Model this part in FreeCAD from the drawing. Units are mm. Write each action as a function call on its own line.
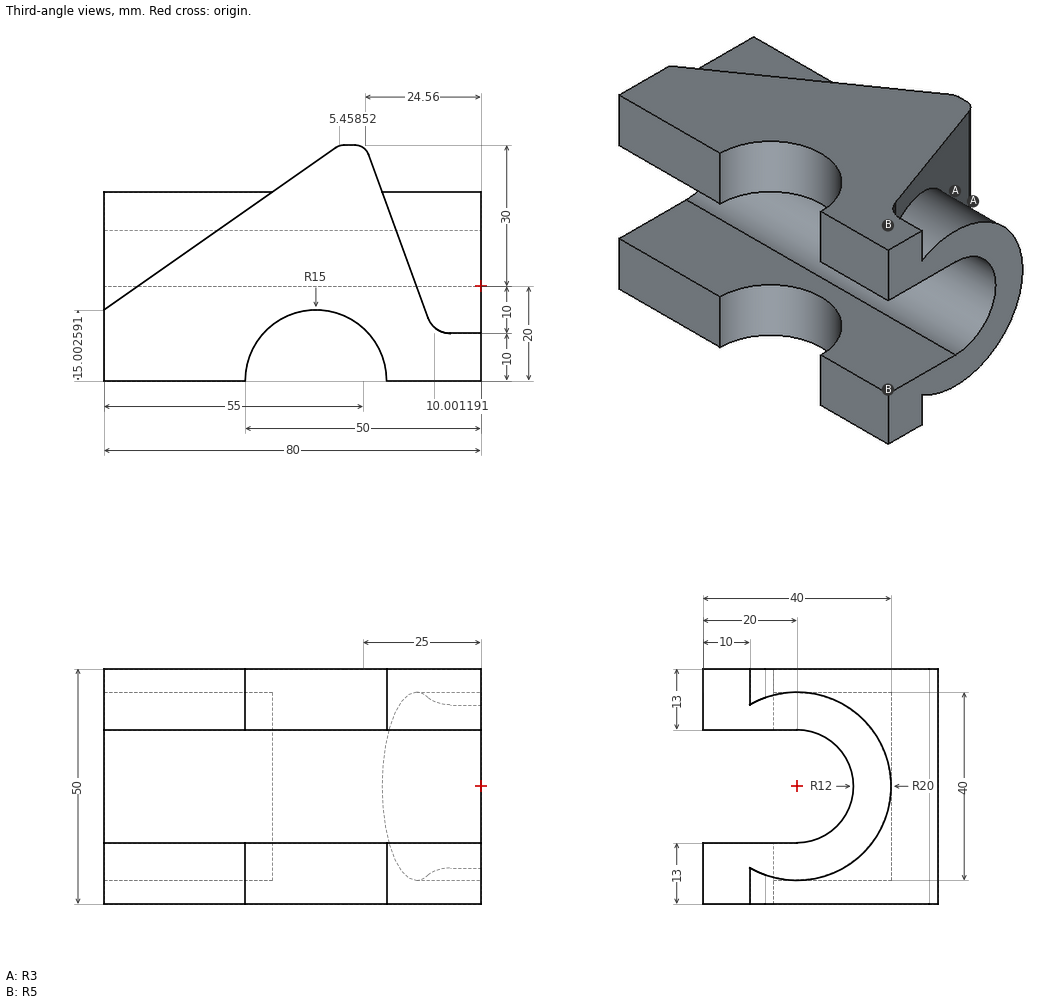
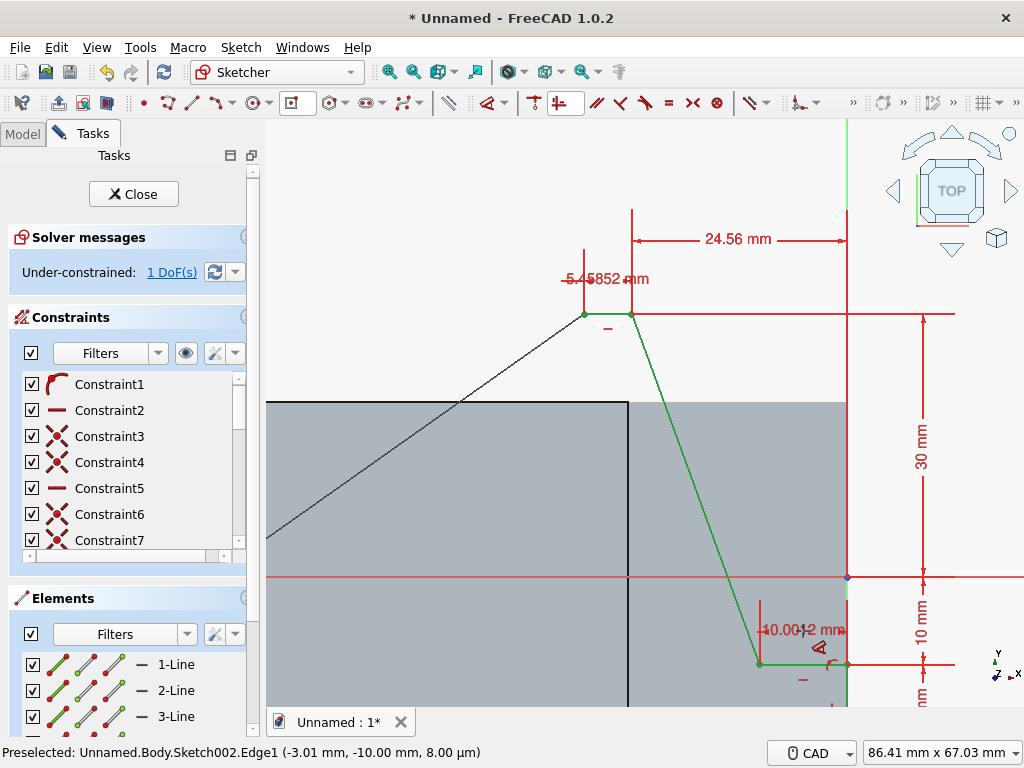
scroll(674, 267, down, 3)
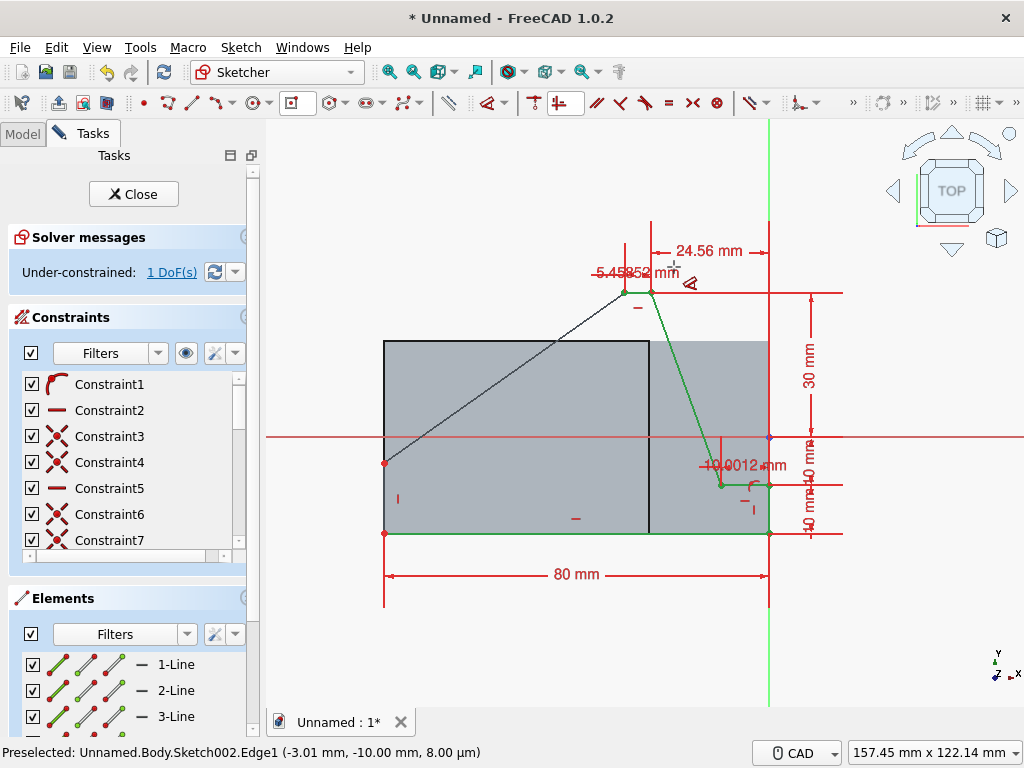
click(384, 484)
click(350, 498)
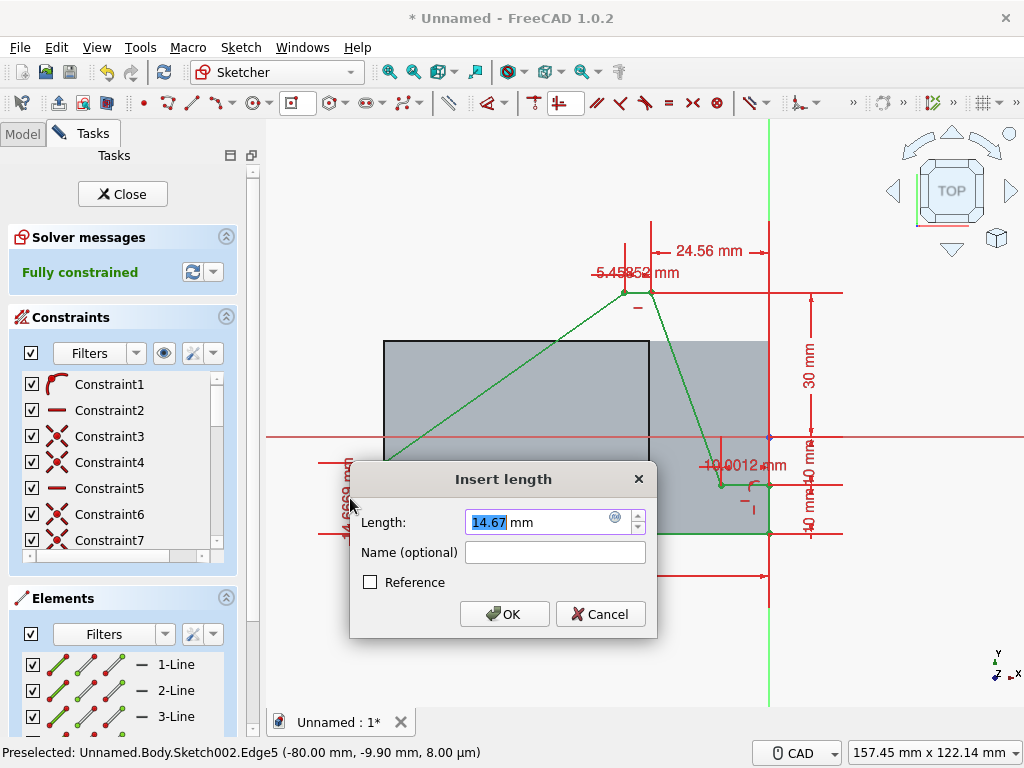
text(15.002591)
key(Return)
key(Escape)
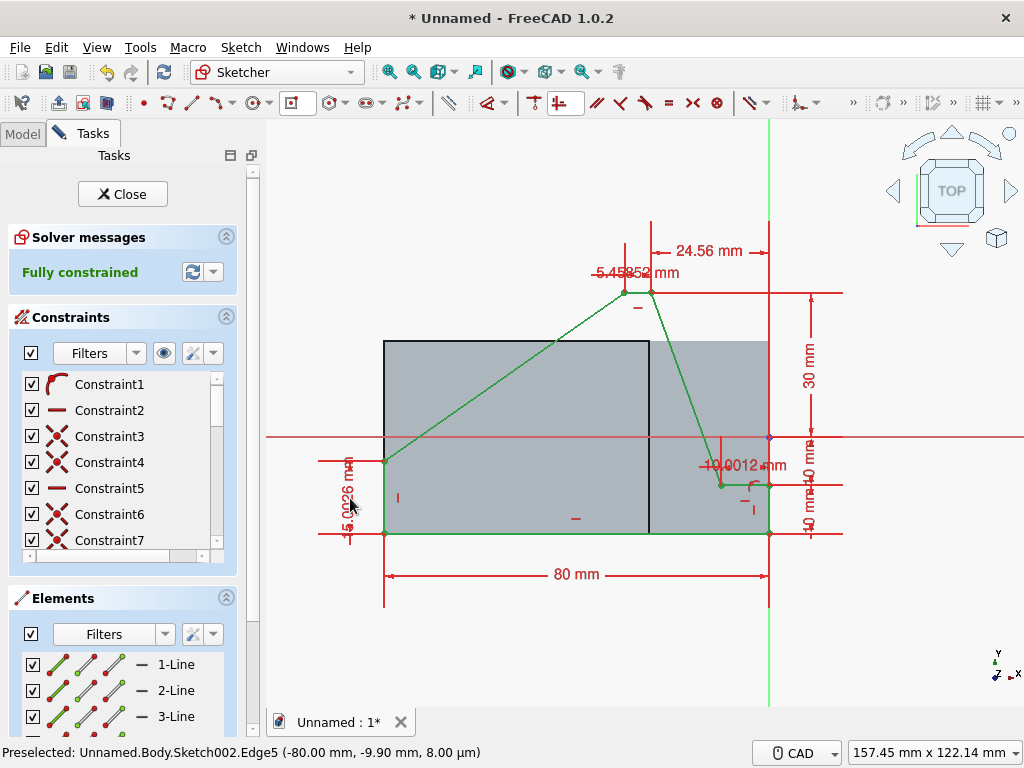
click(123, 194)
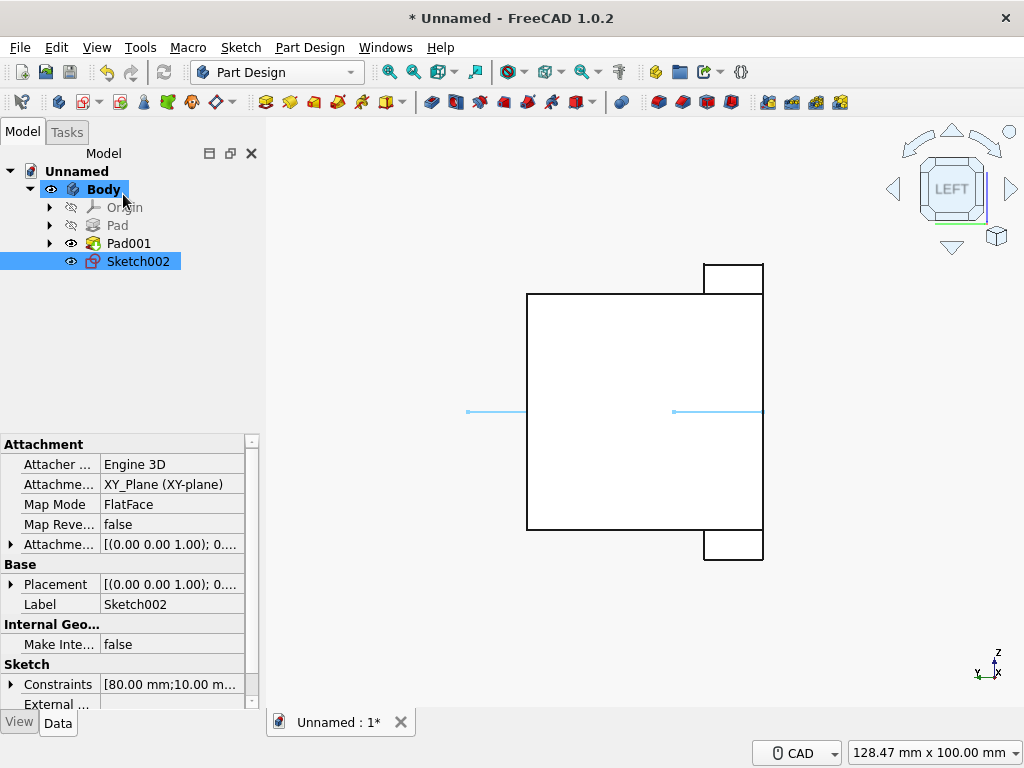
click(266, 102)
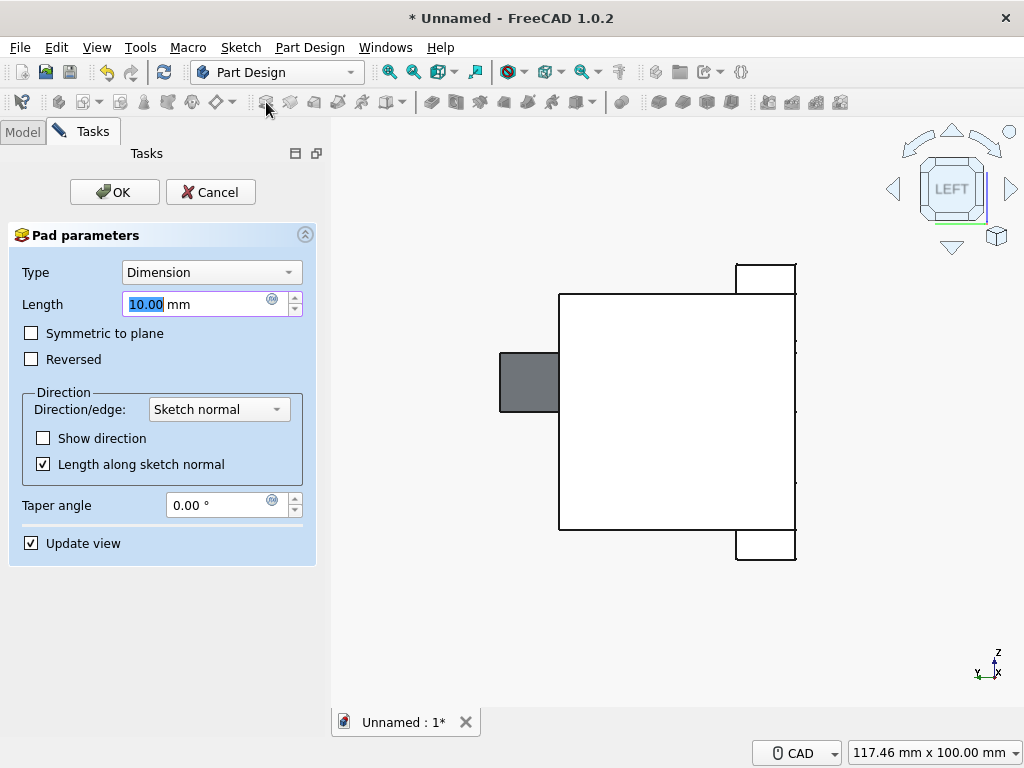
text(50)
key(Tab)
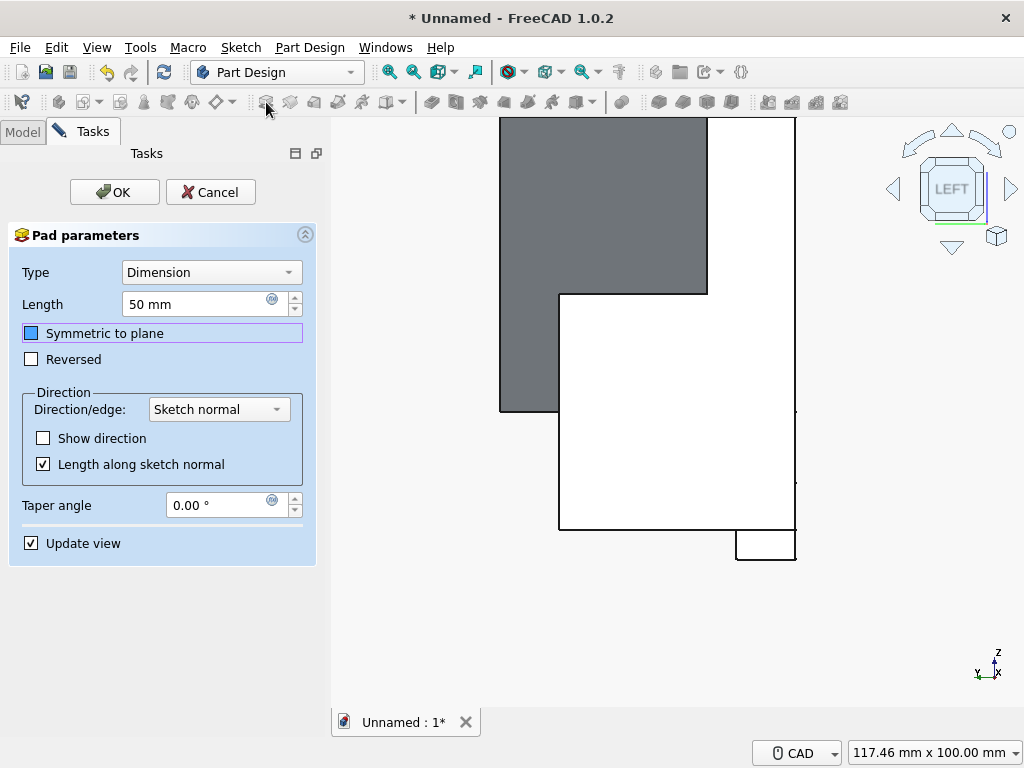
click(30, 333)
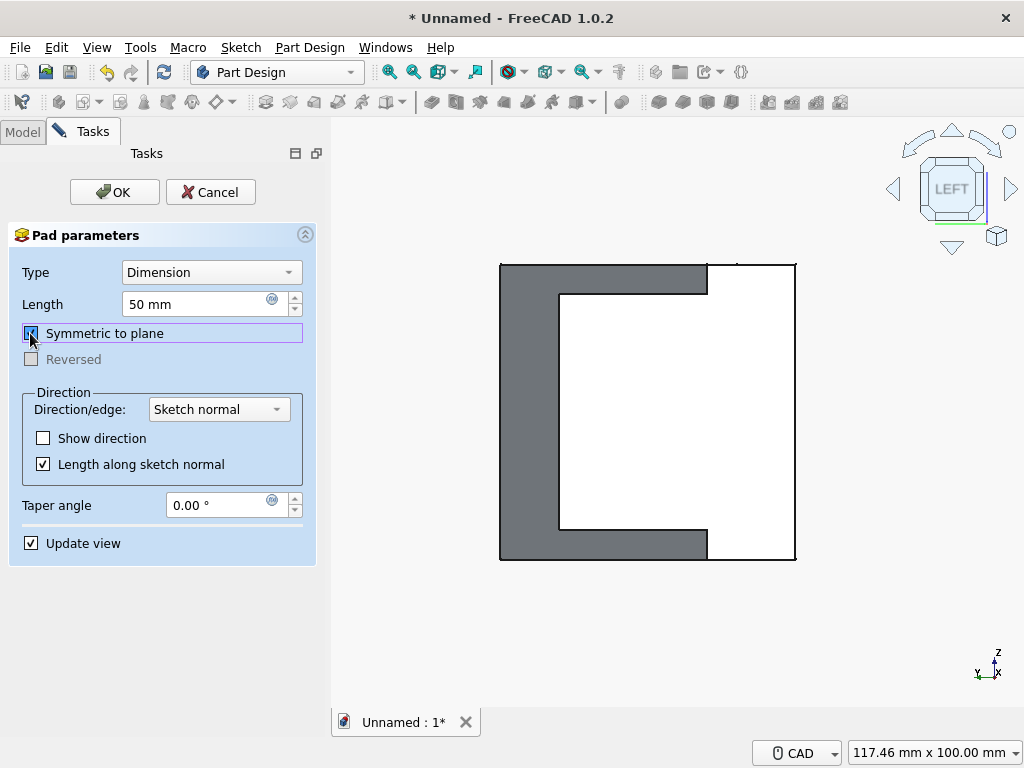
click(115, 192)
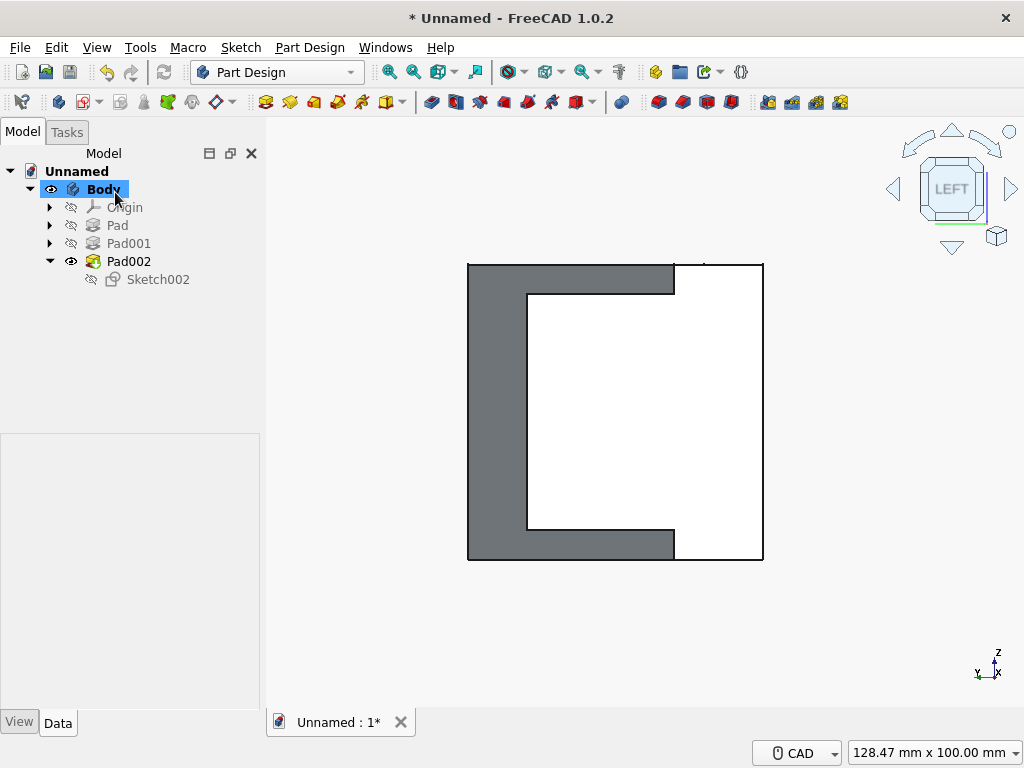
key(0)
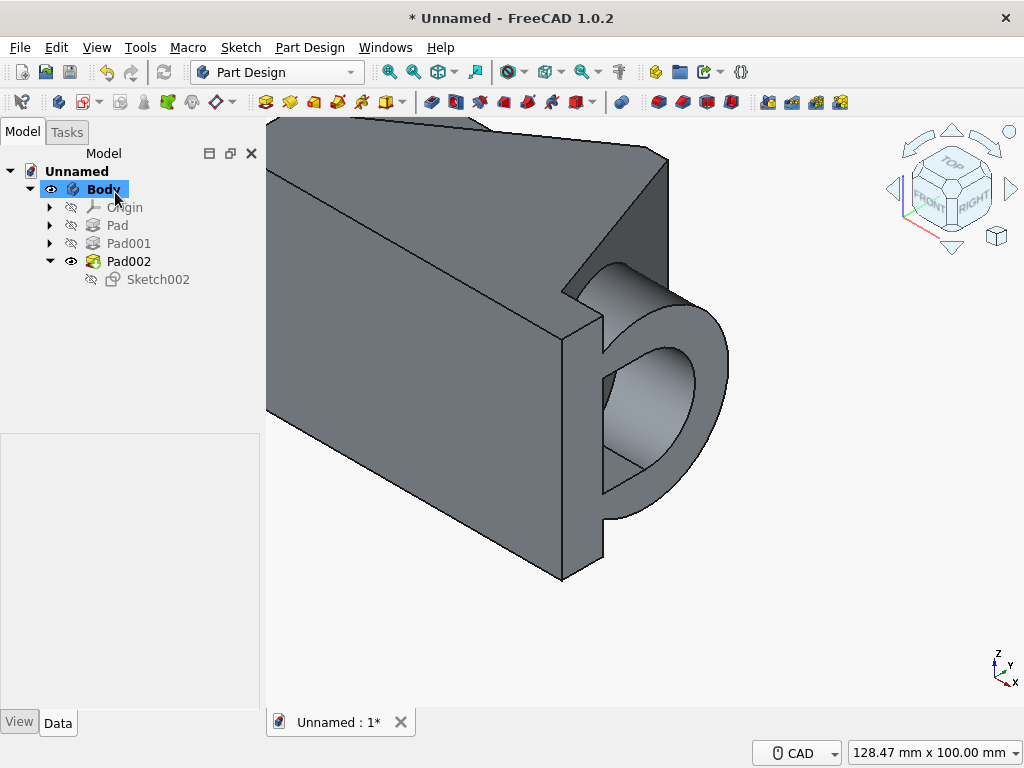
click(390, 72)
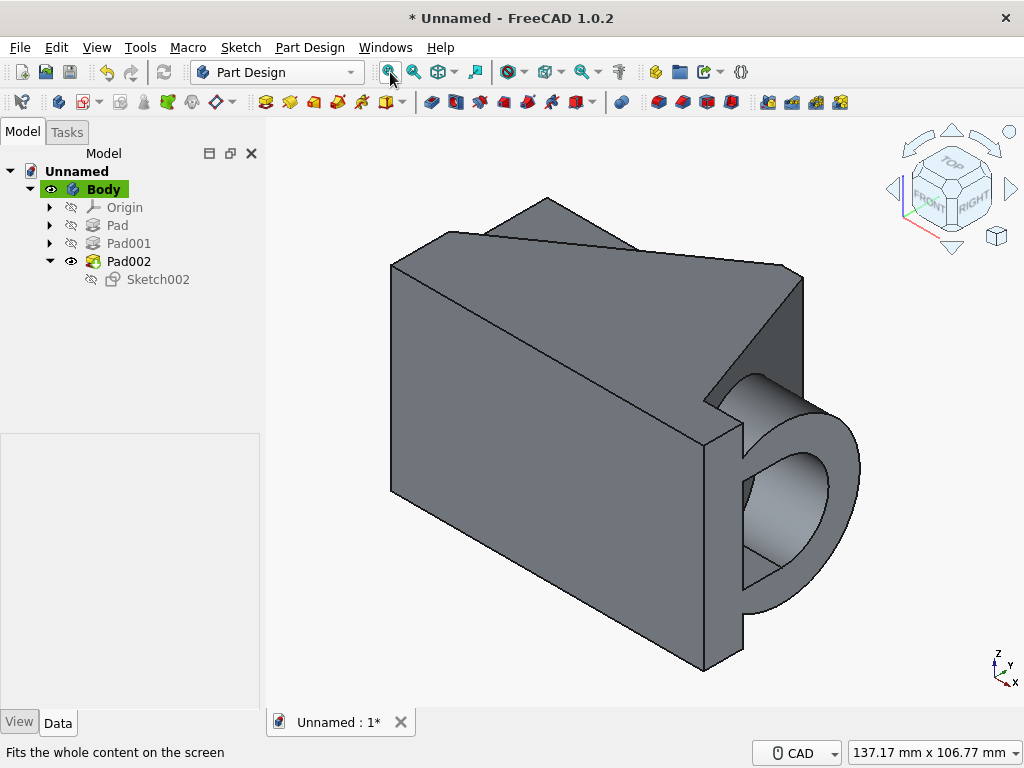
key(2)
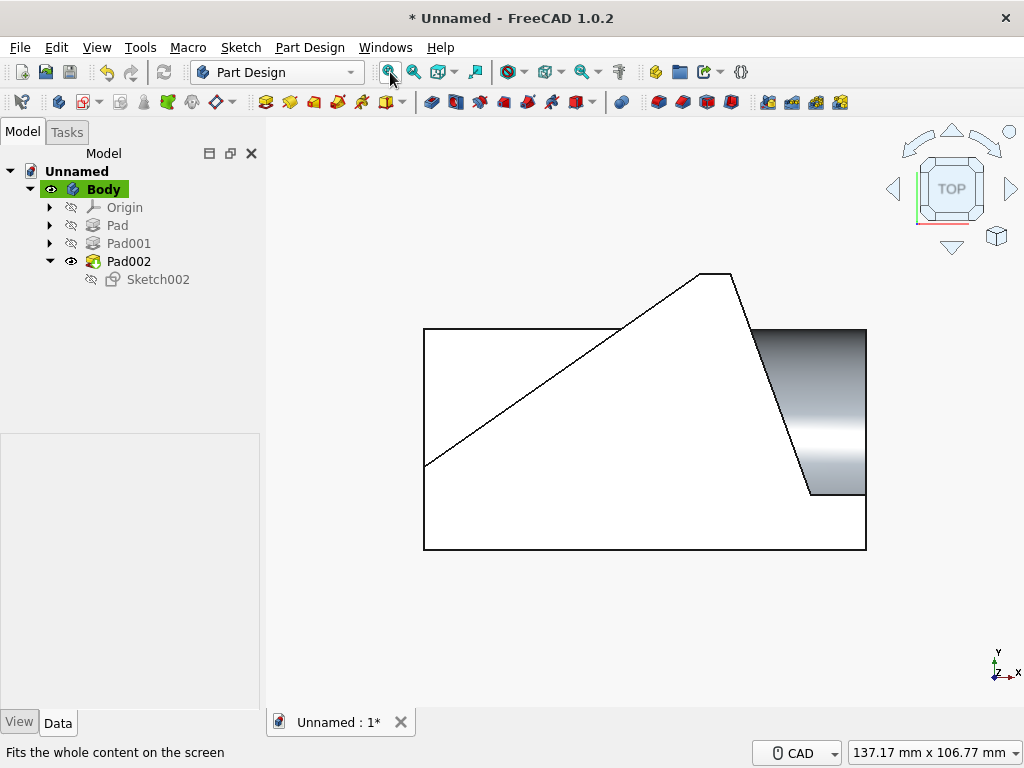
key(1)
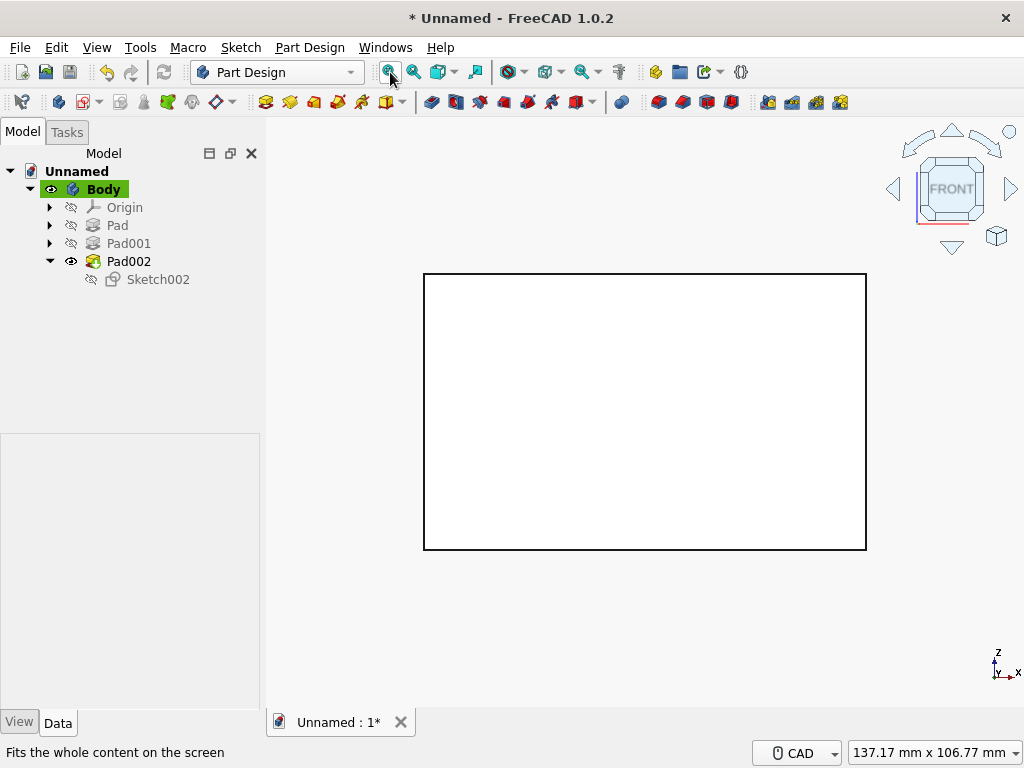
key(3)